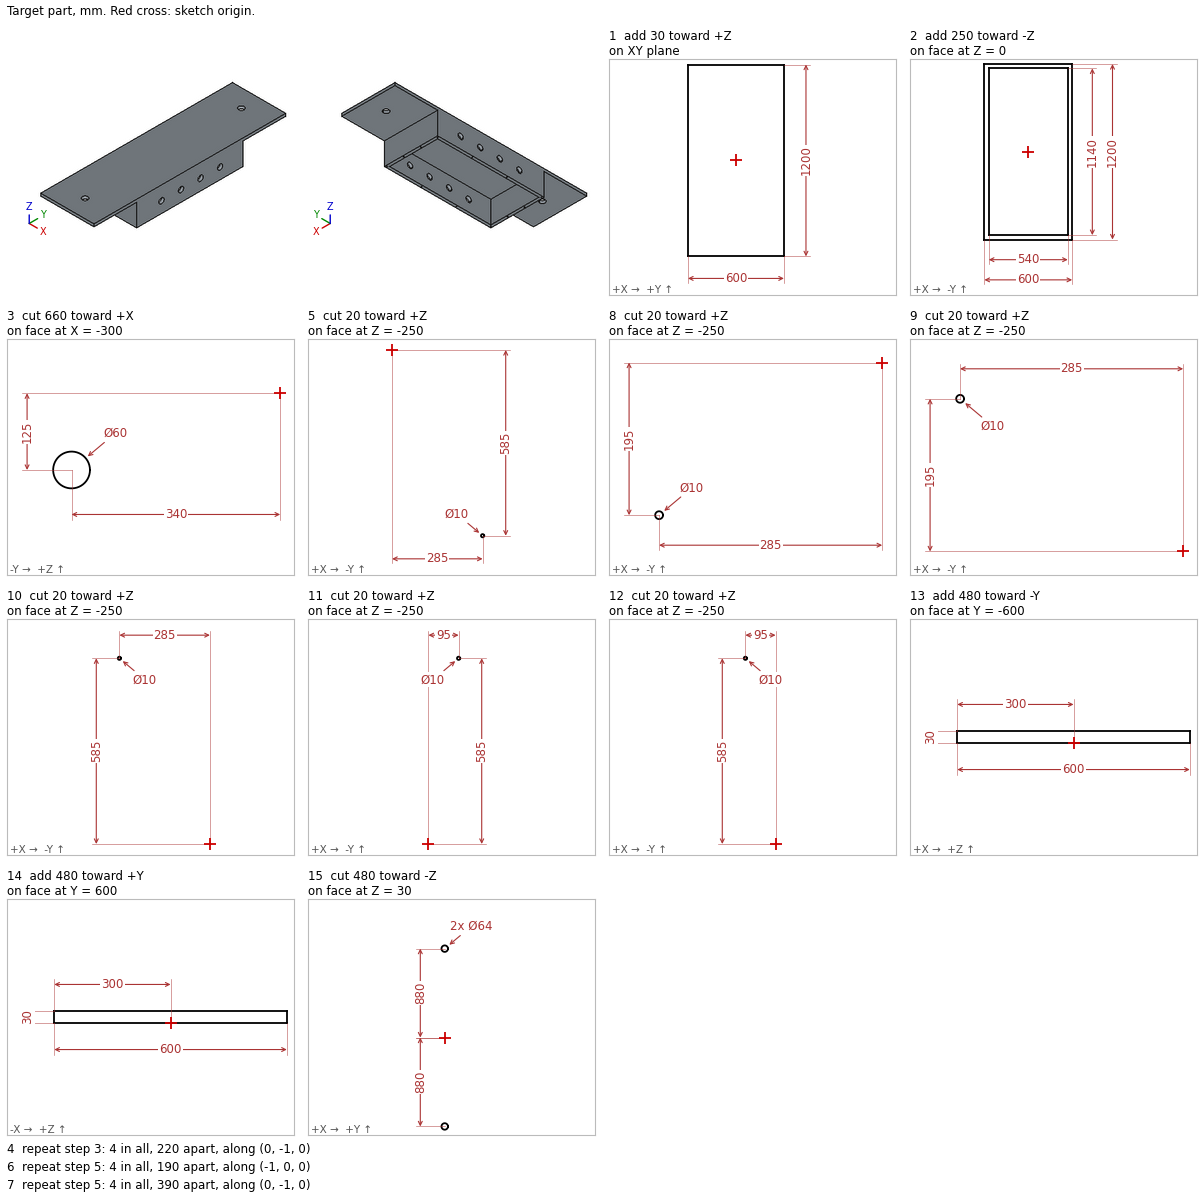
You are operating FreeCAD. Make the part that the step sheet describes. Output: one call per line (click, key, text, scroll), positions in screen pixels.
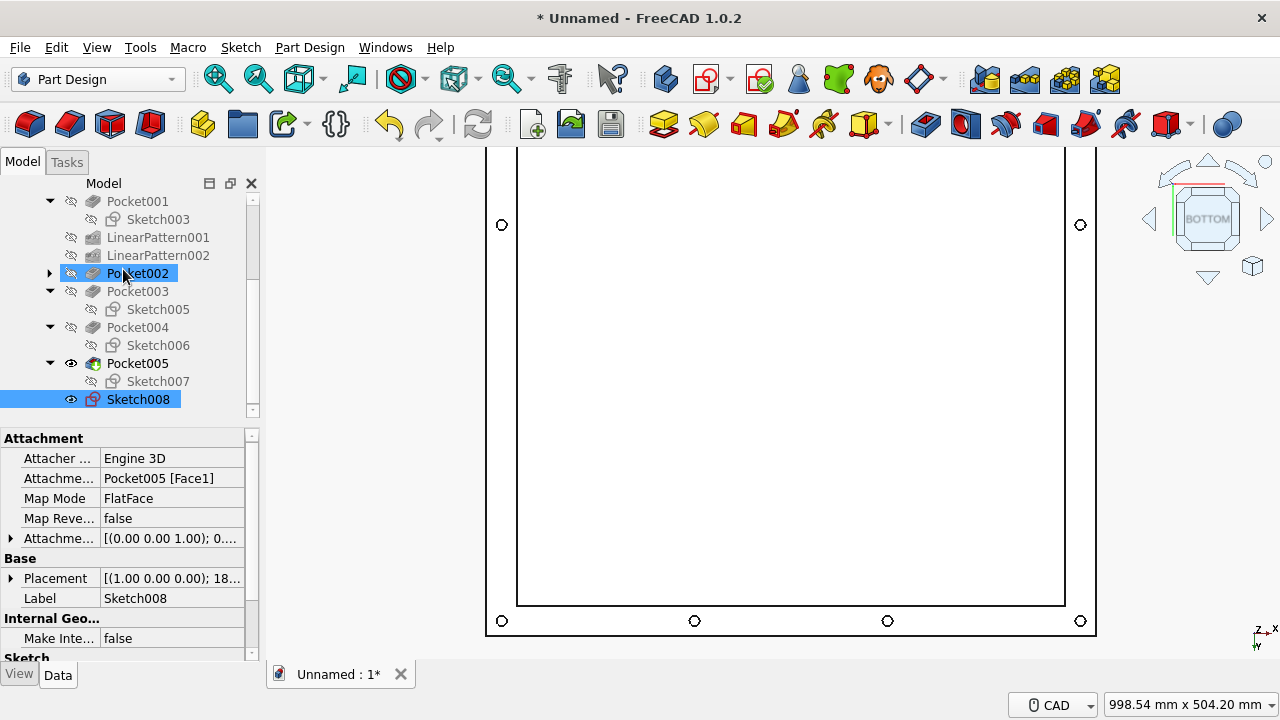
click(926, 124)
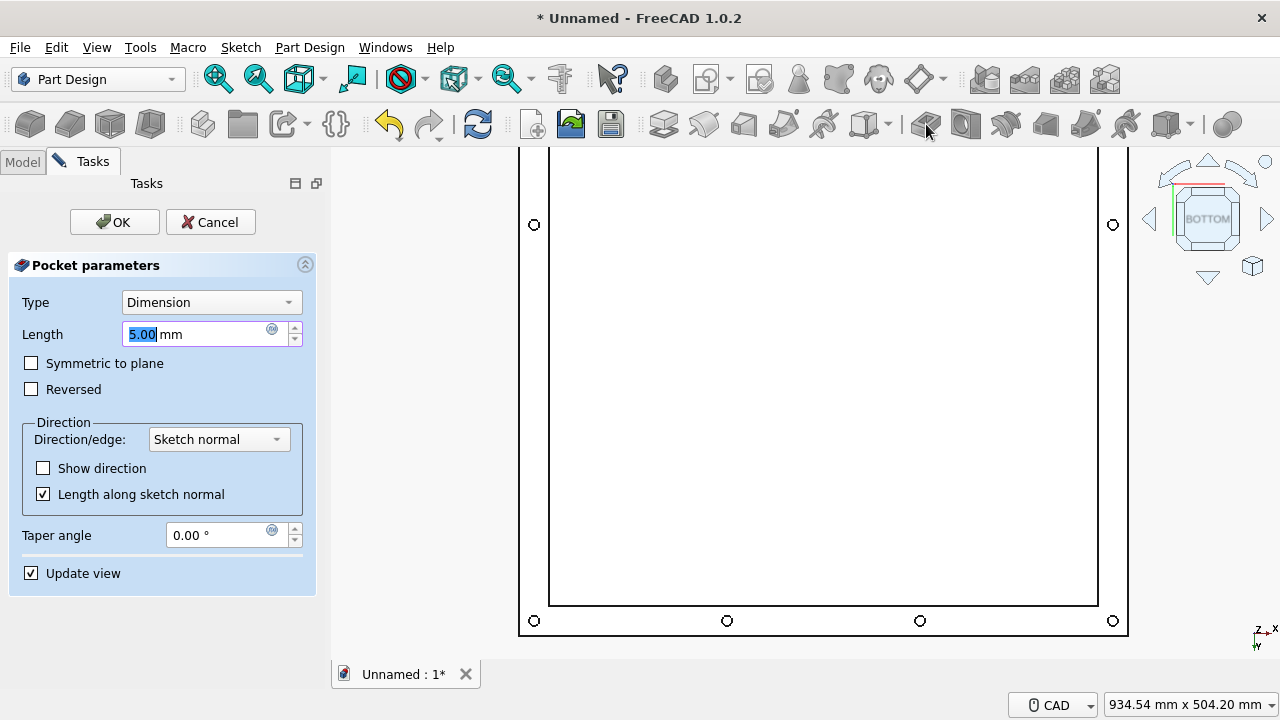
text(20)
key(Tab)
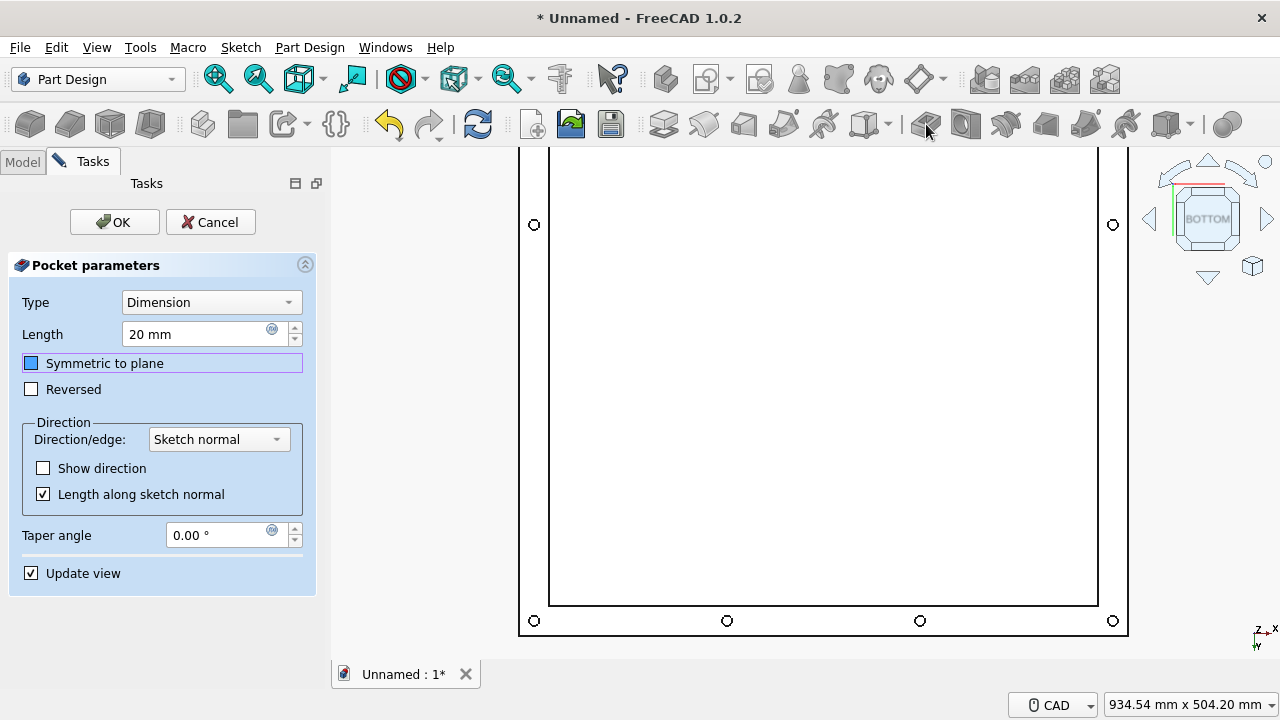
click(115, 222)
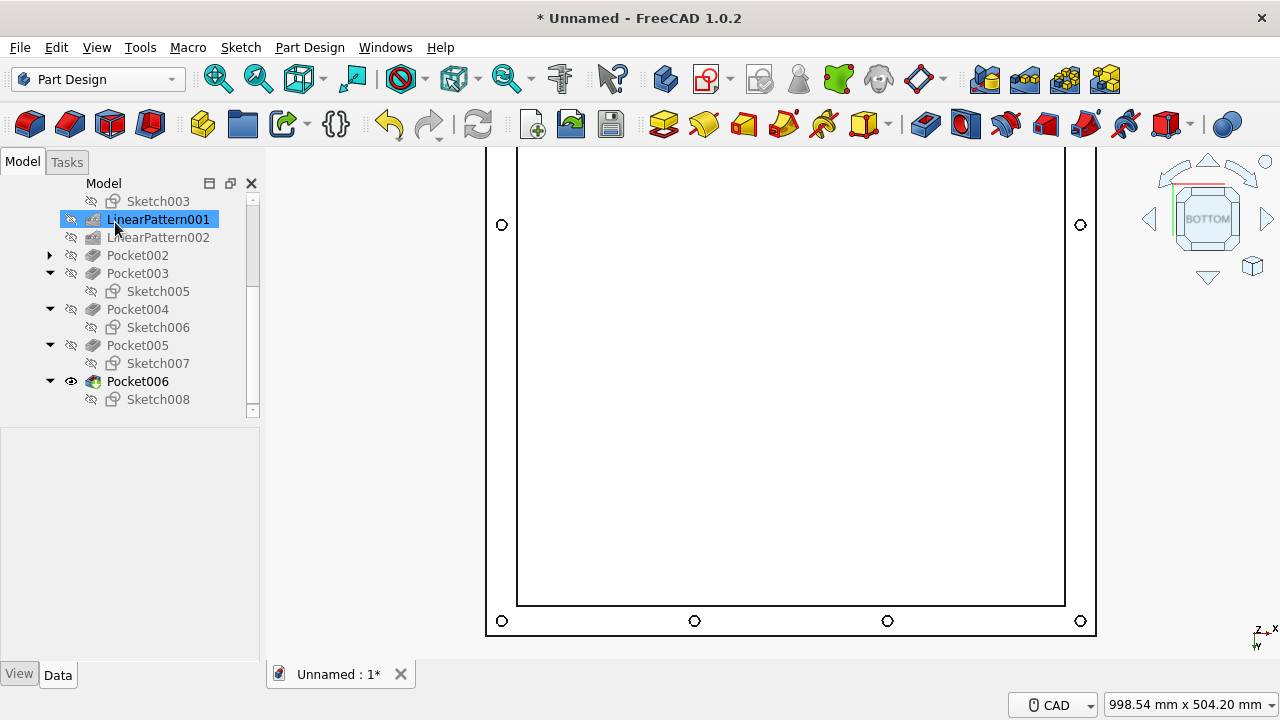
click(220, 80)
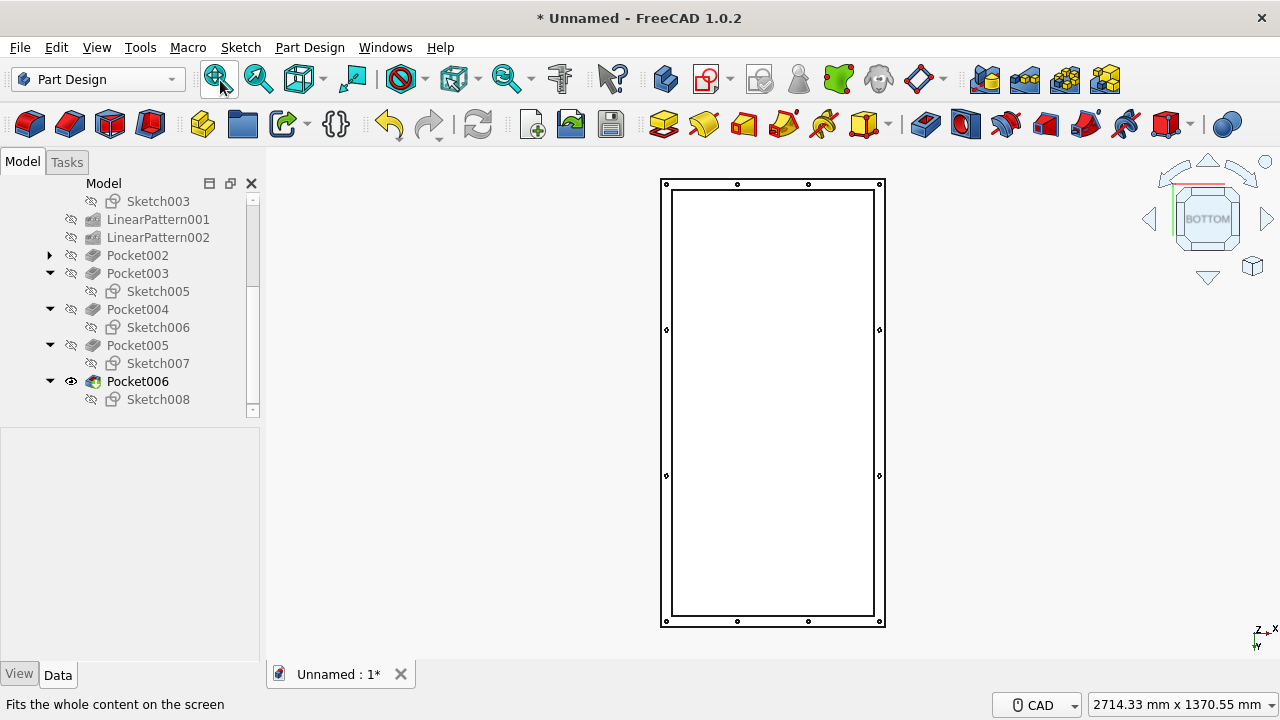
key(0)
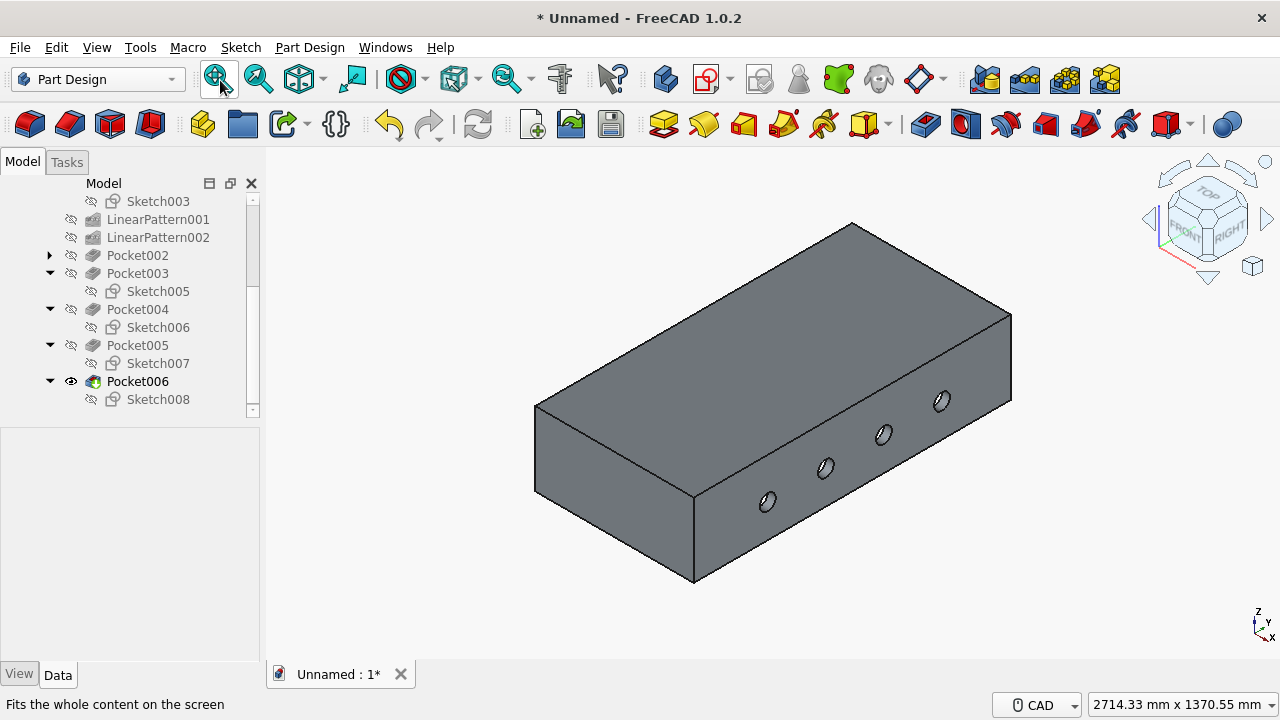
click(637, 507)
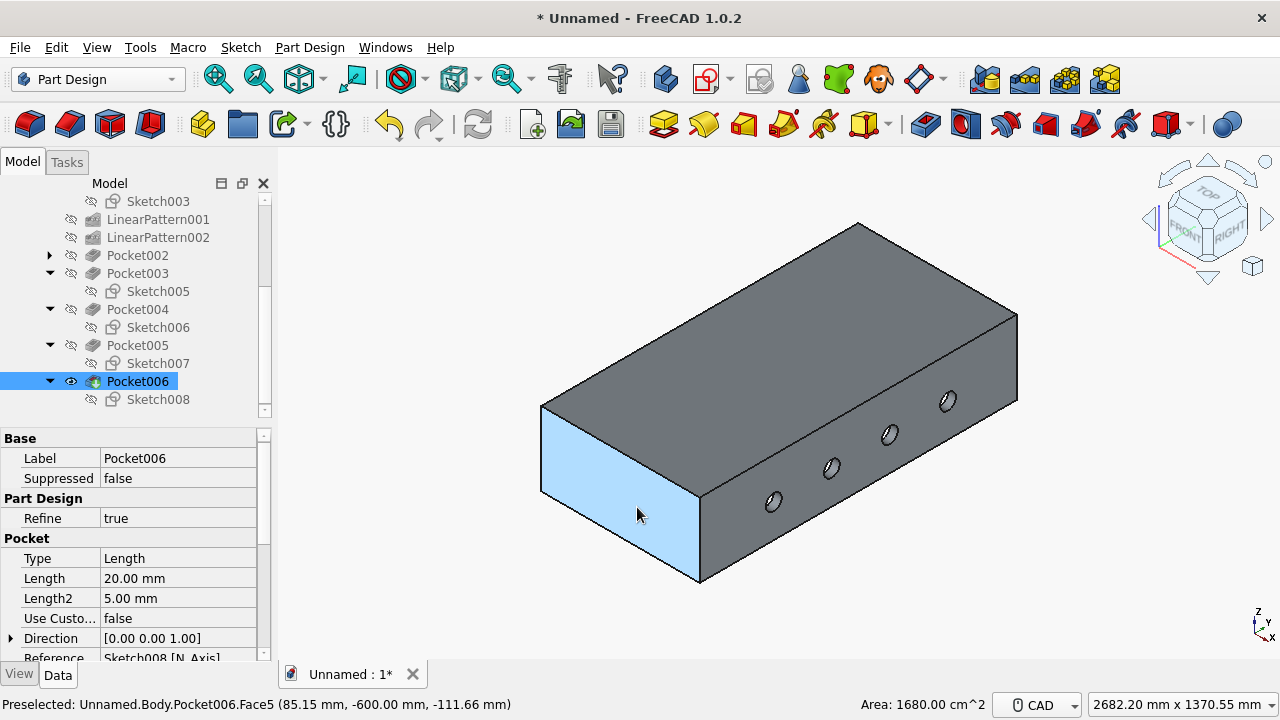
click(706, 80)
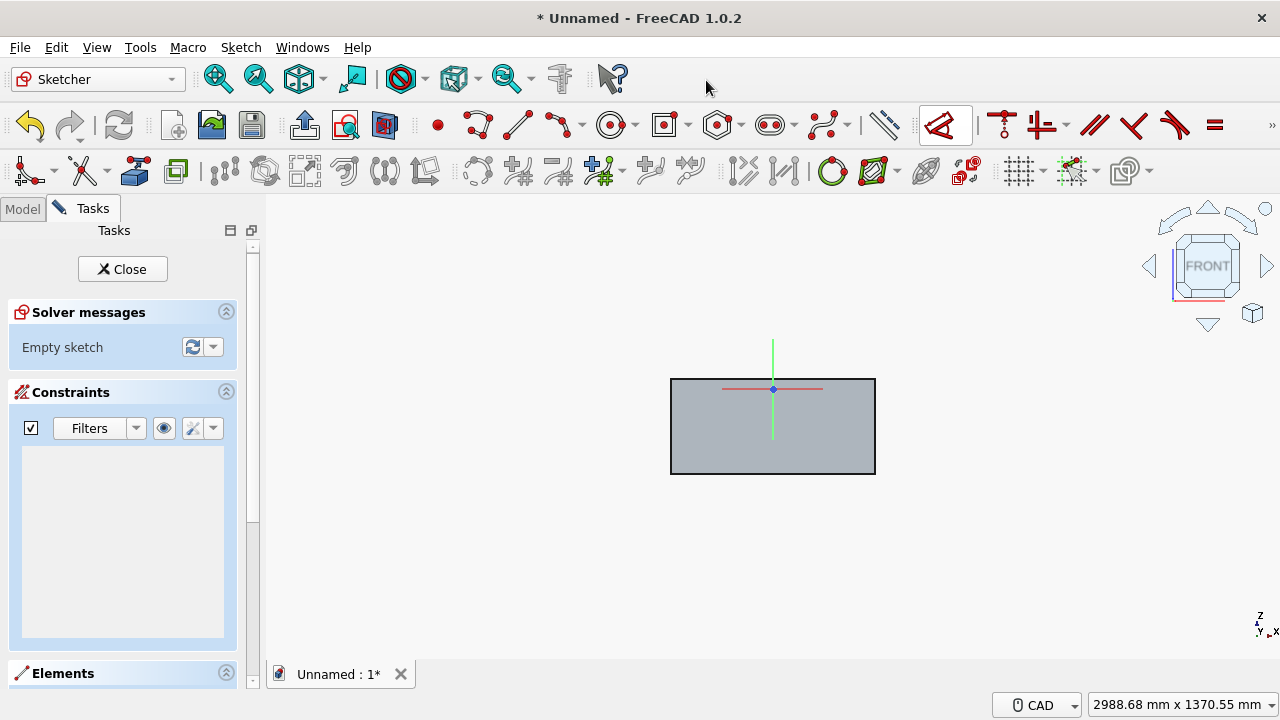
scroll(813, 359, up, 5)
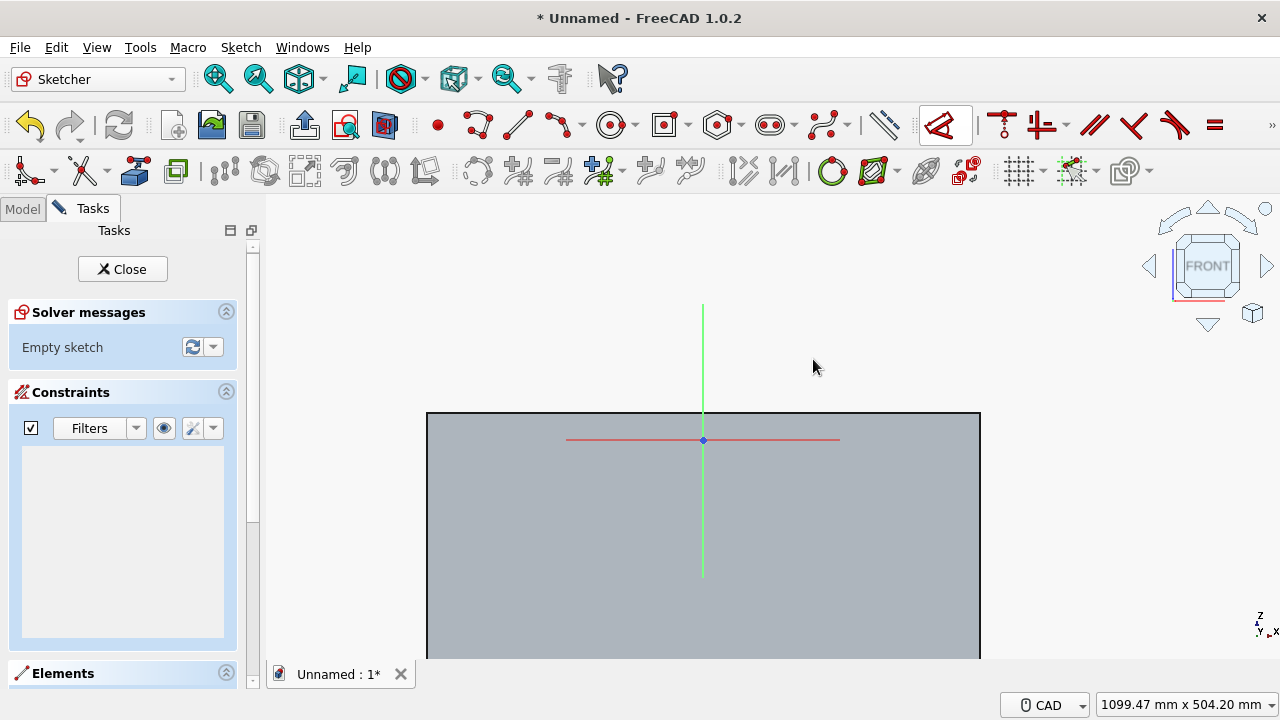
click(690, 126)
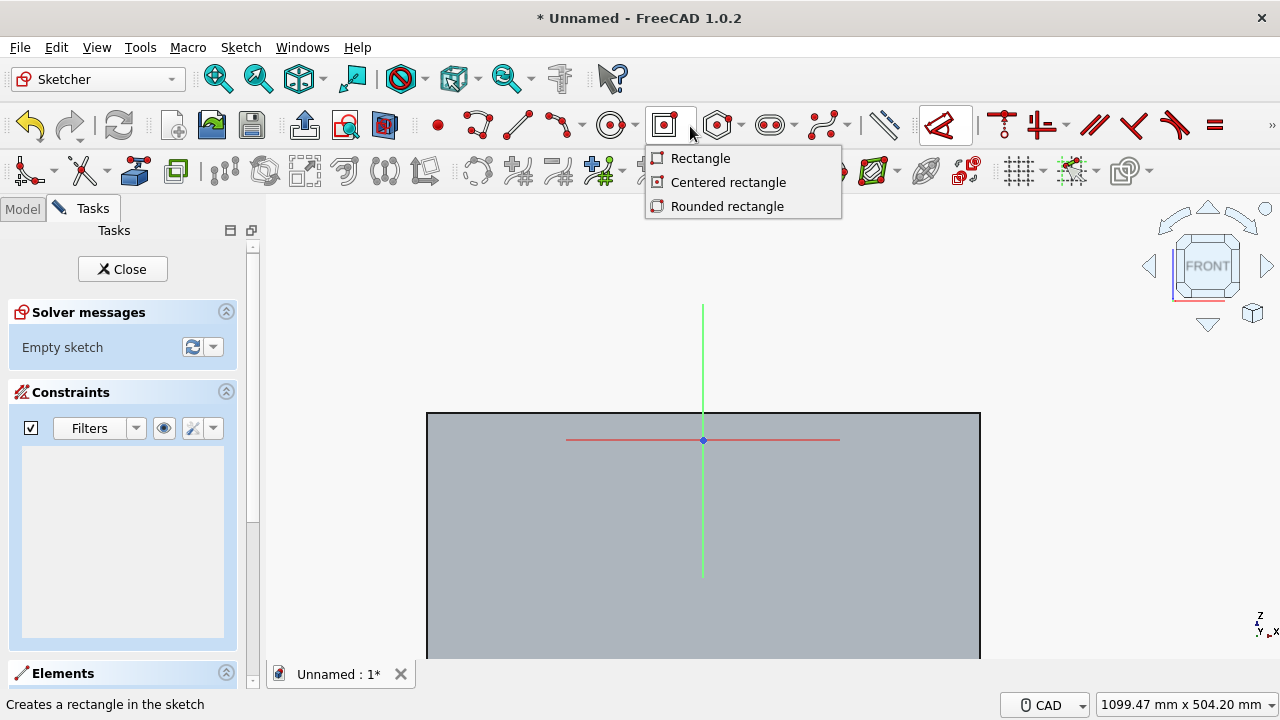
click(744, 158)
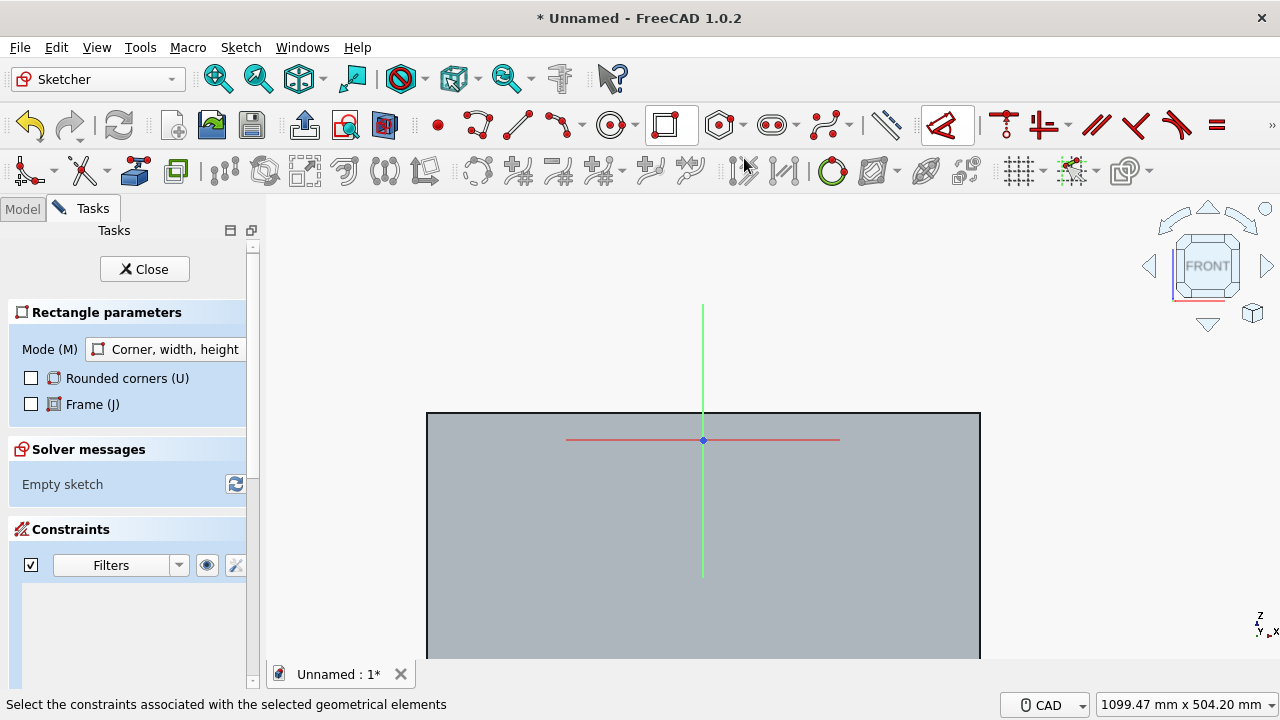
click(427, 413)
click(980, 440)
key(Escape)